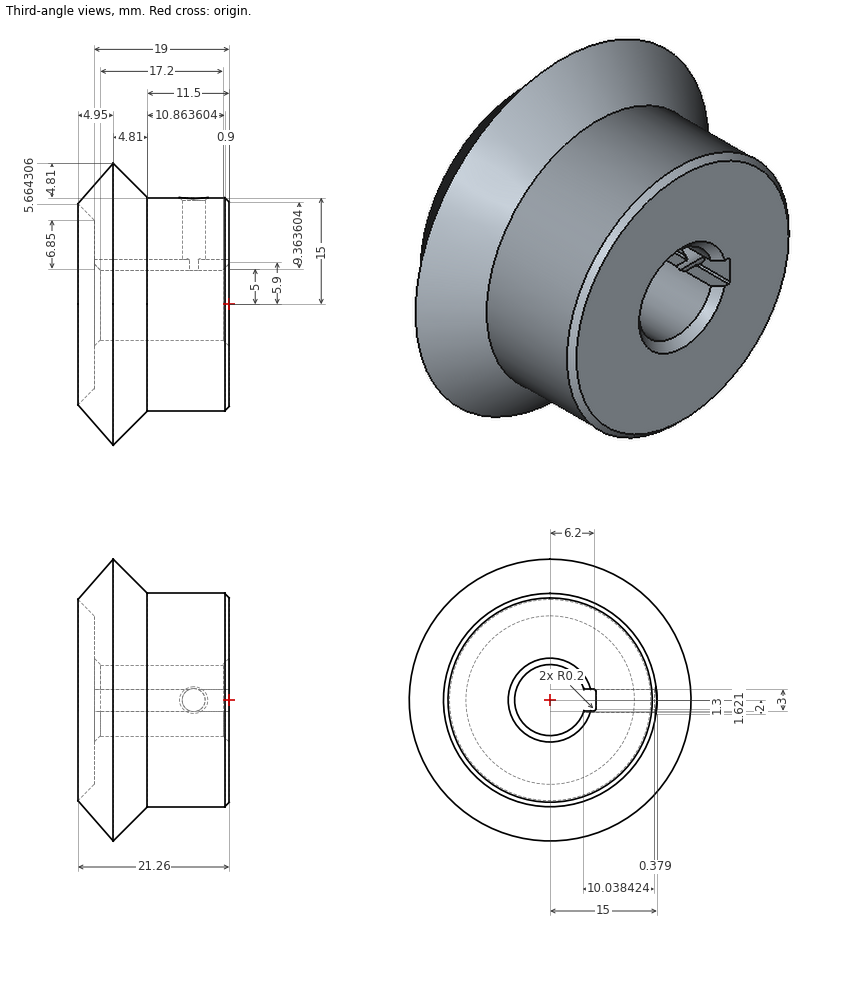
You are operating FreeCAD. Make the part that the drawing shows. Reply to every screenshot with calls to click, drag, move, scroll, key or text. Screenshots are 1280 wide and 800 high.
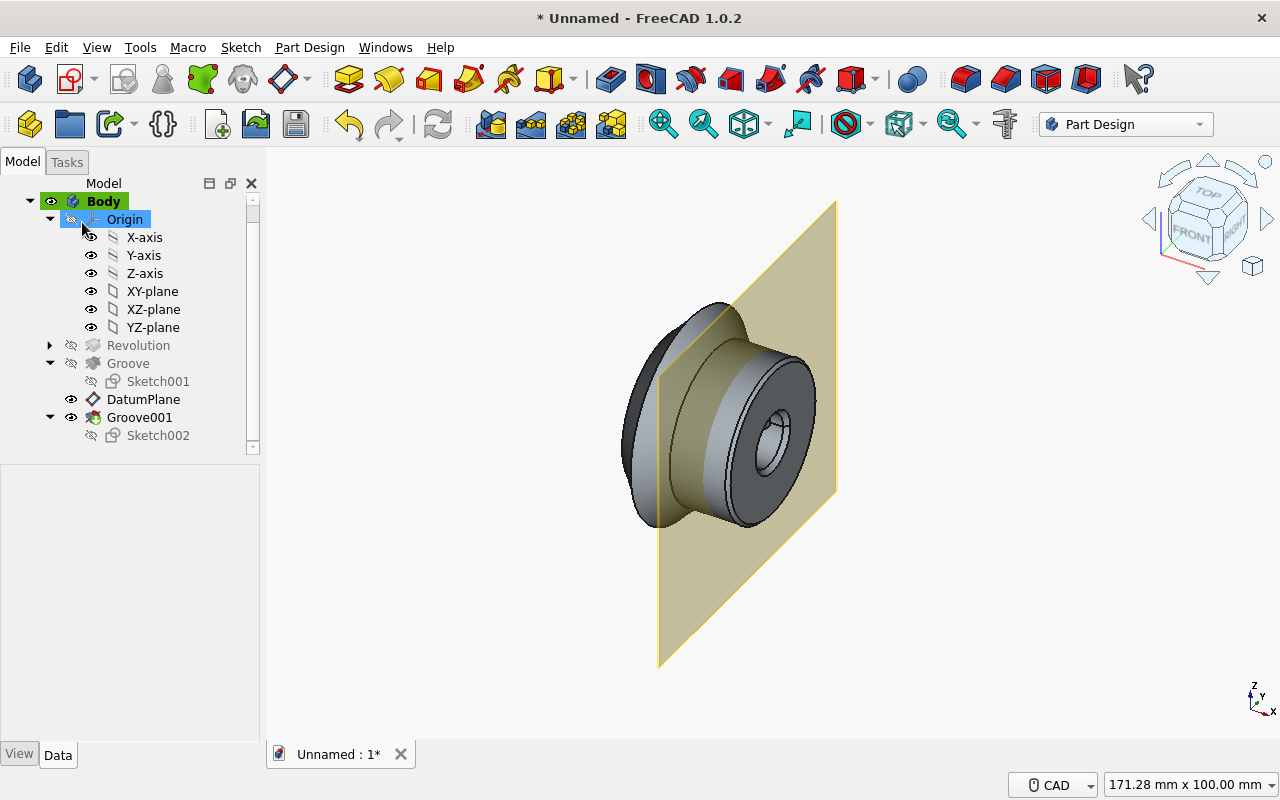
click(116, 399)
key(space)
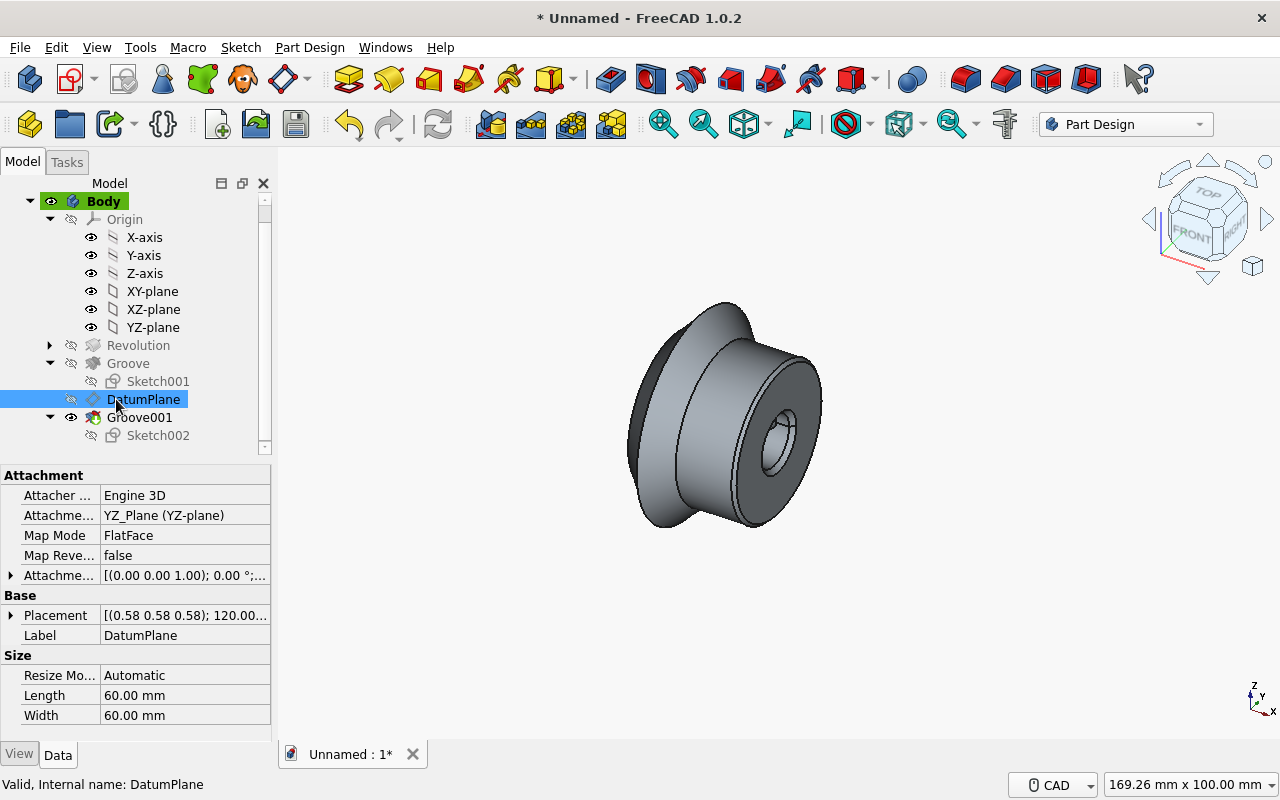
click(318, 699)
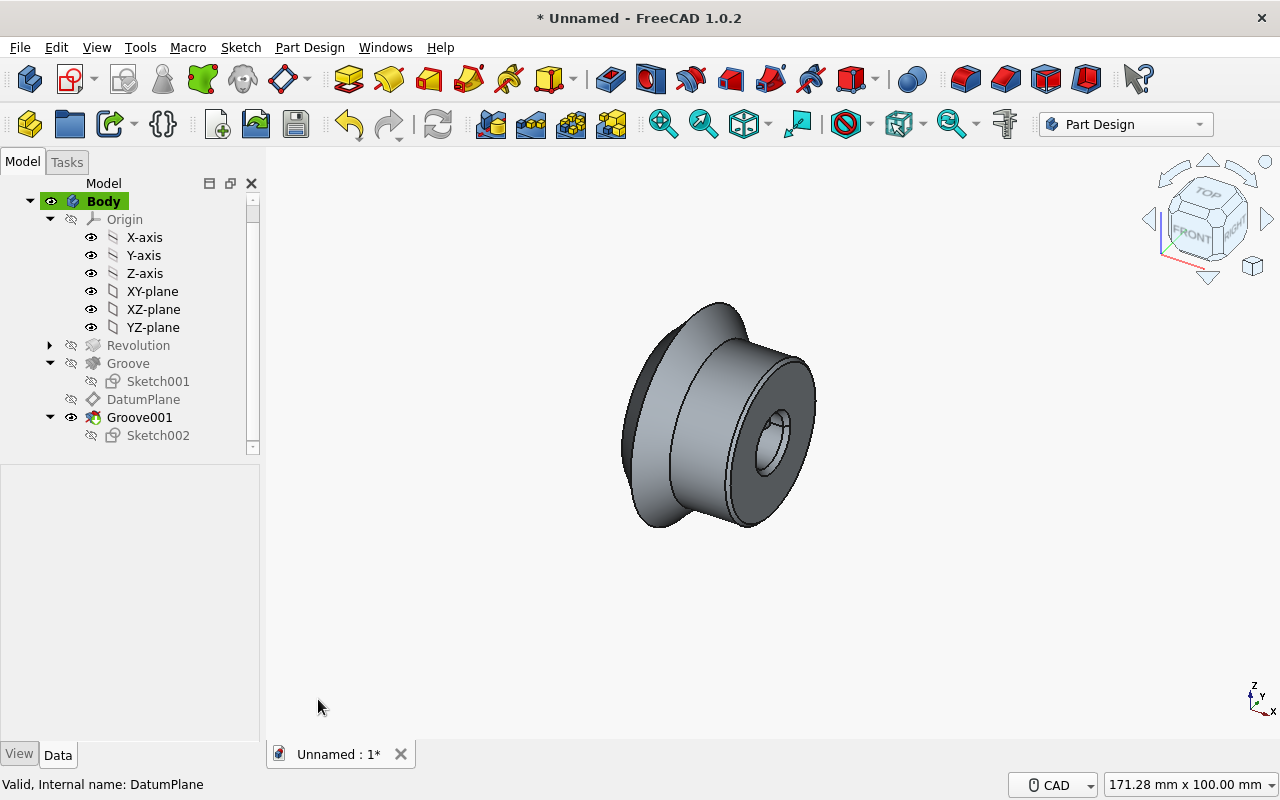
click(70, 80)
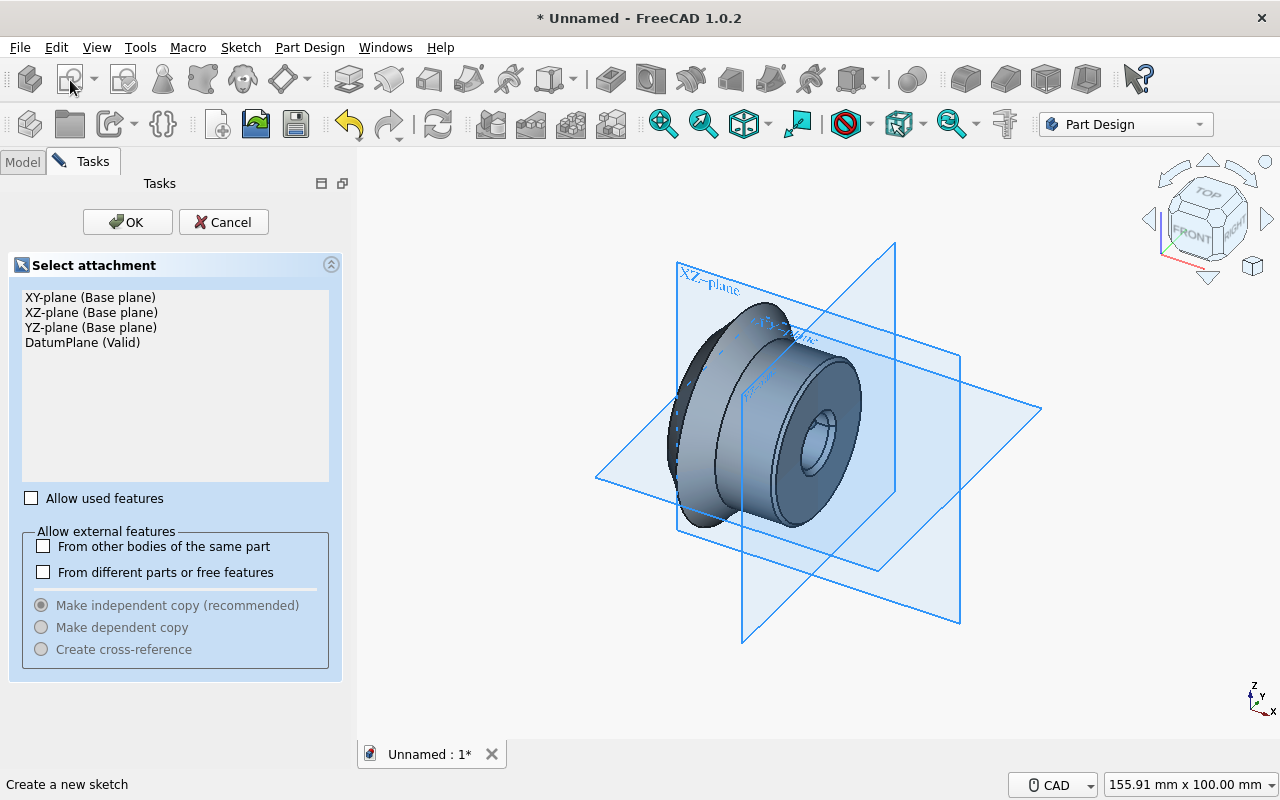
click(82, 328)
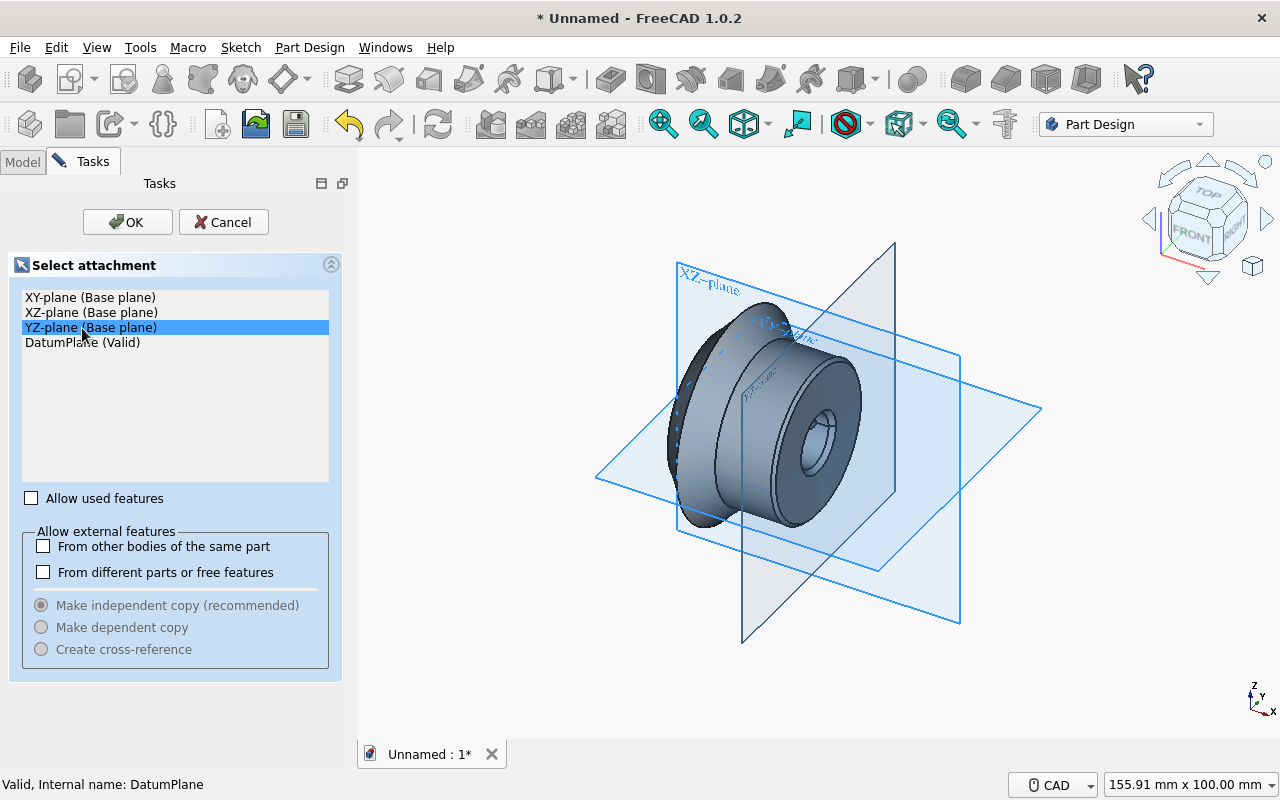
click(128, 222)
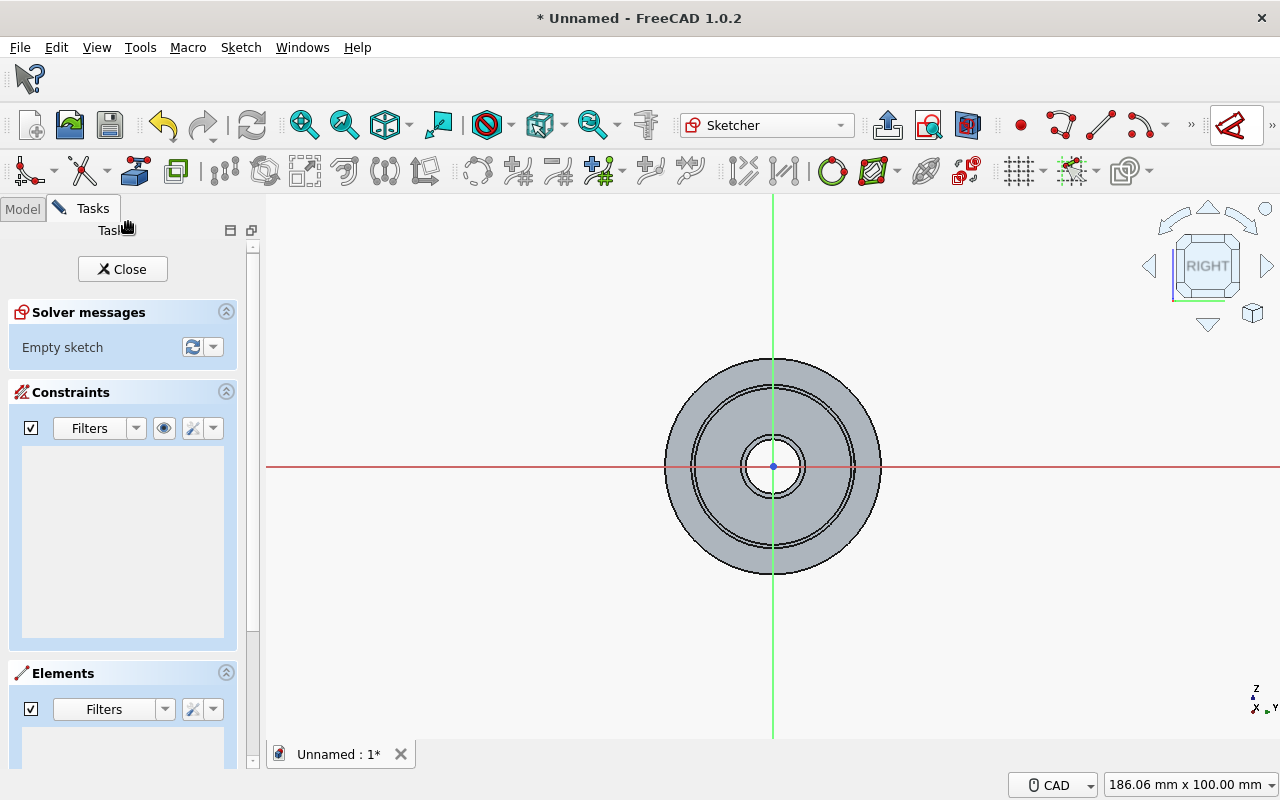
scroll(796, 466, up, 14)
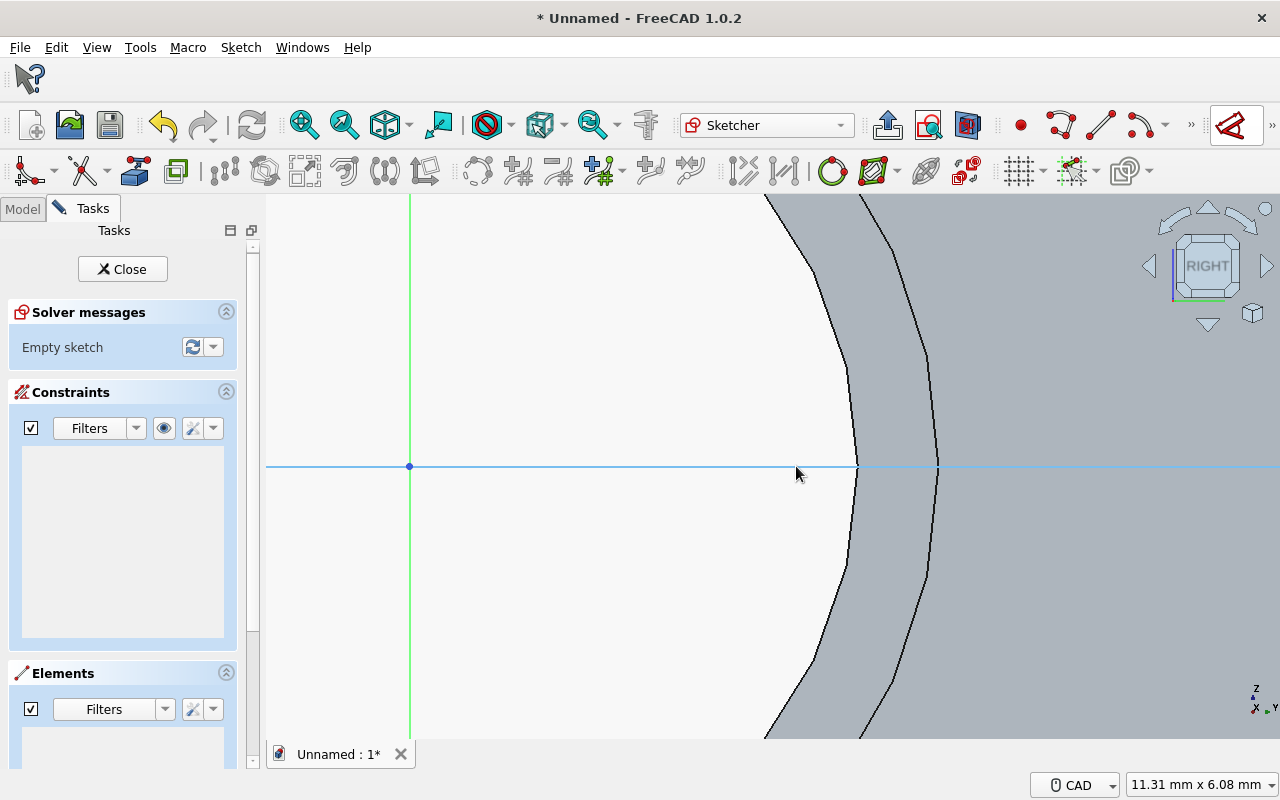
click(1102, 126)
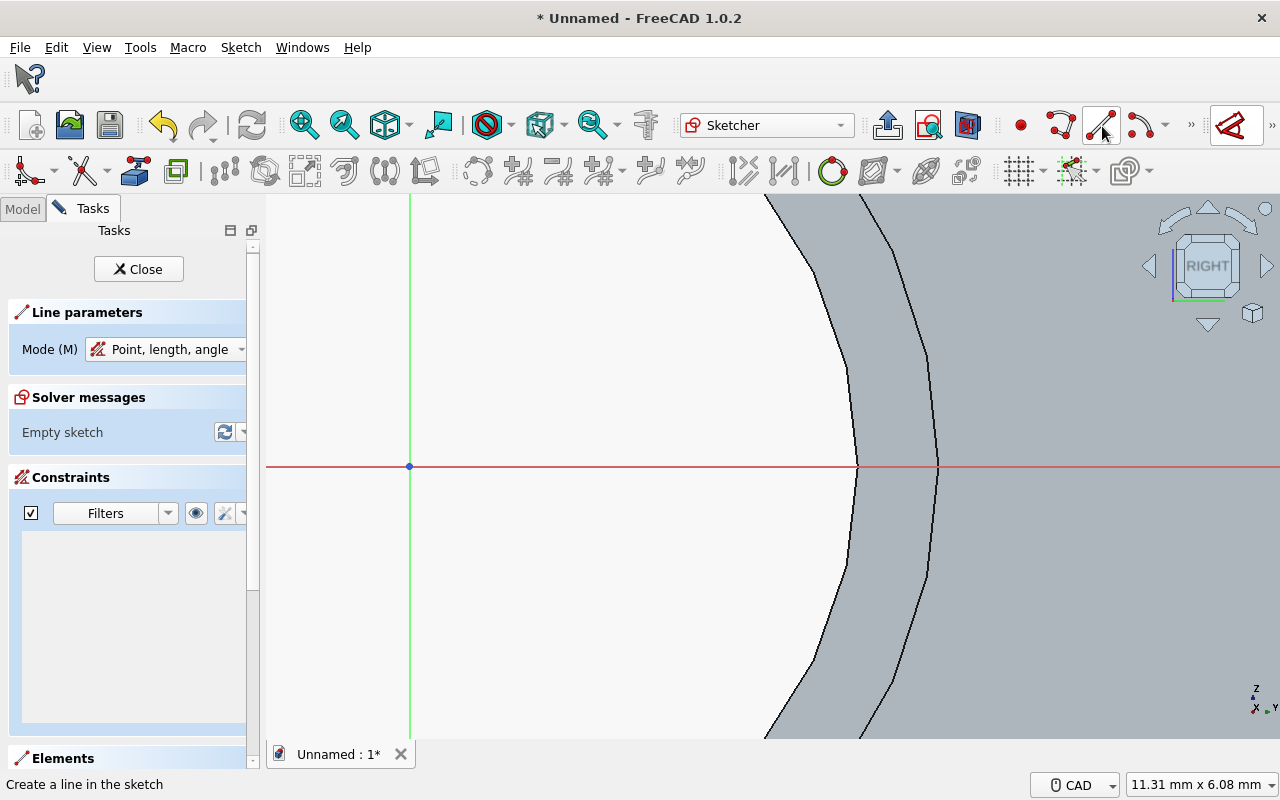
click(983, 583)
click(983, 350)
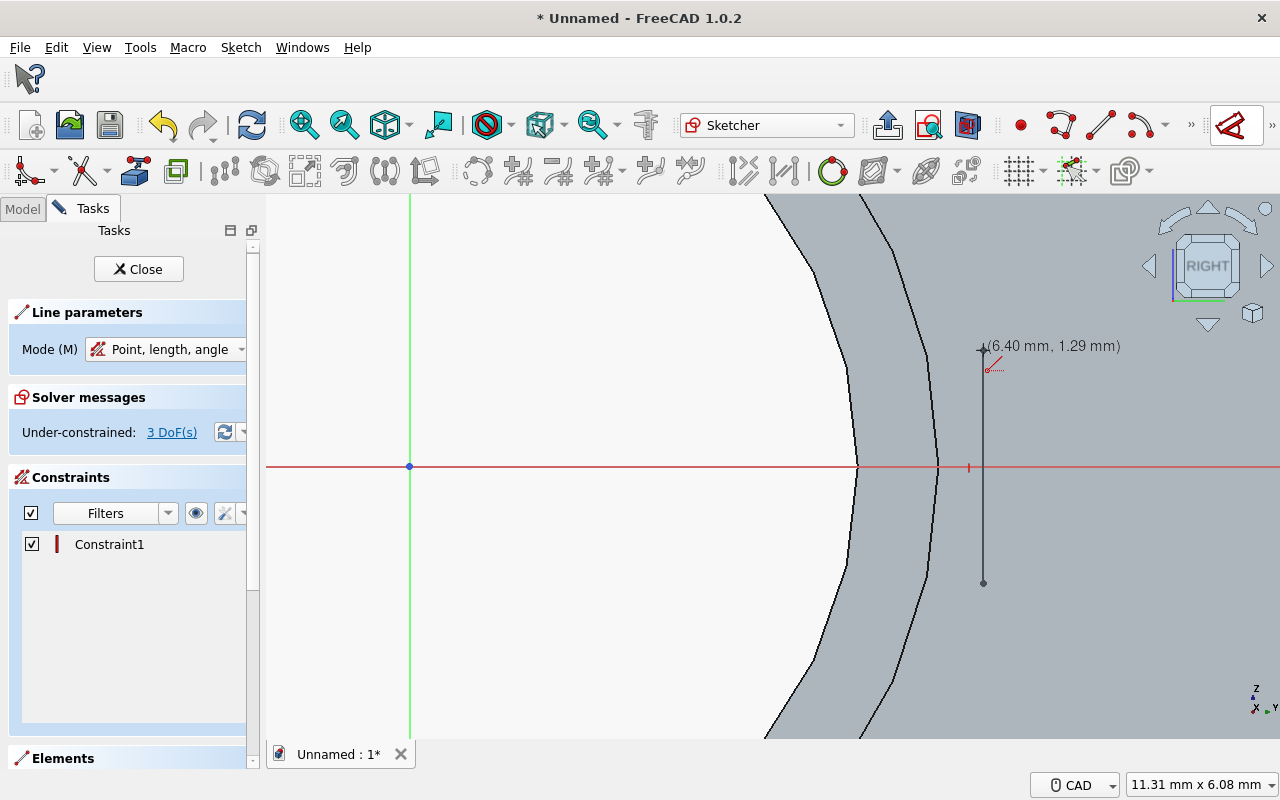
click(1062, 126)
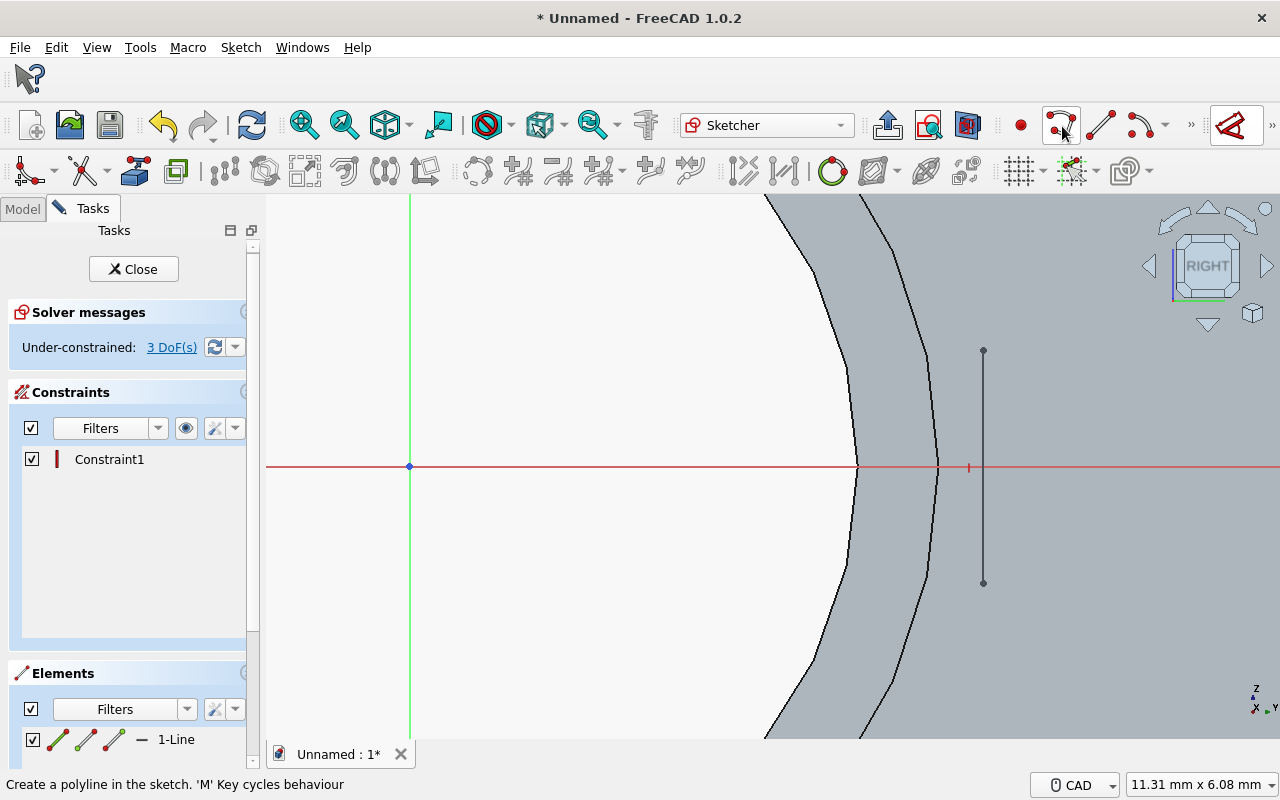
click(965, 332)
click(410, 332)
click(419, 601)
click(965, 601)
right_click(965, 601)